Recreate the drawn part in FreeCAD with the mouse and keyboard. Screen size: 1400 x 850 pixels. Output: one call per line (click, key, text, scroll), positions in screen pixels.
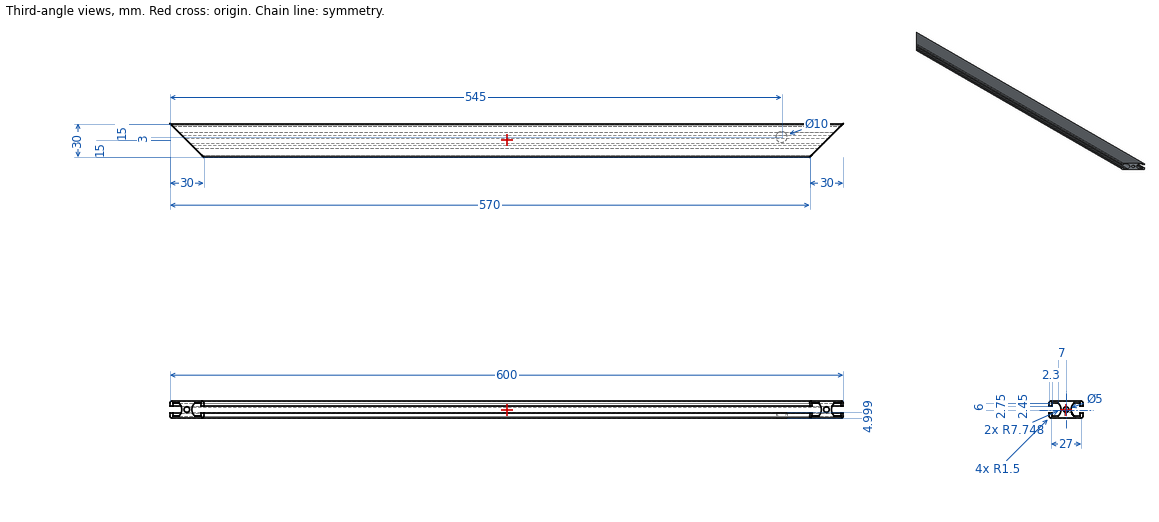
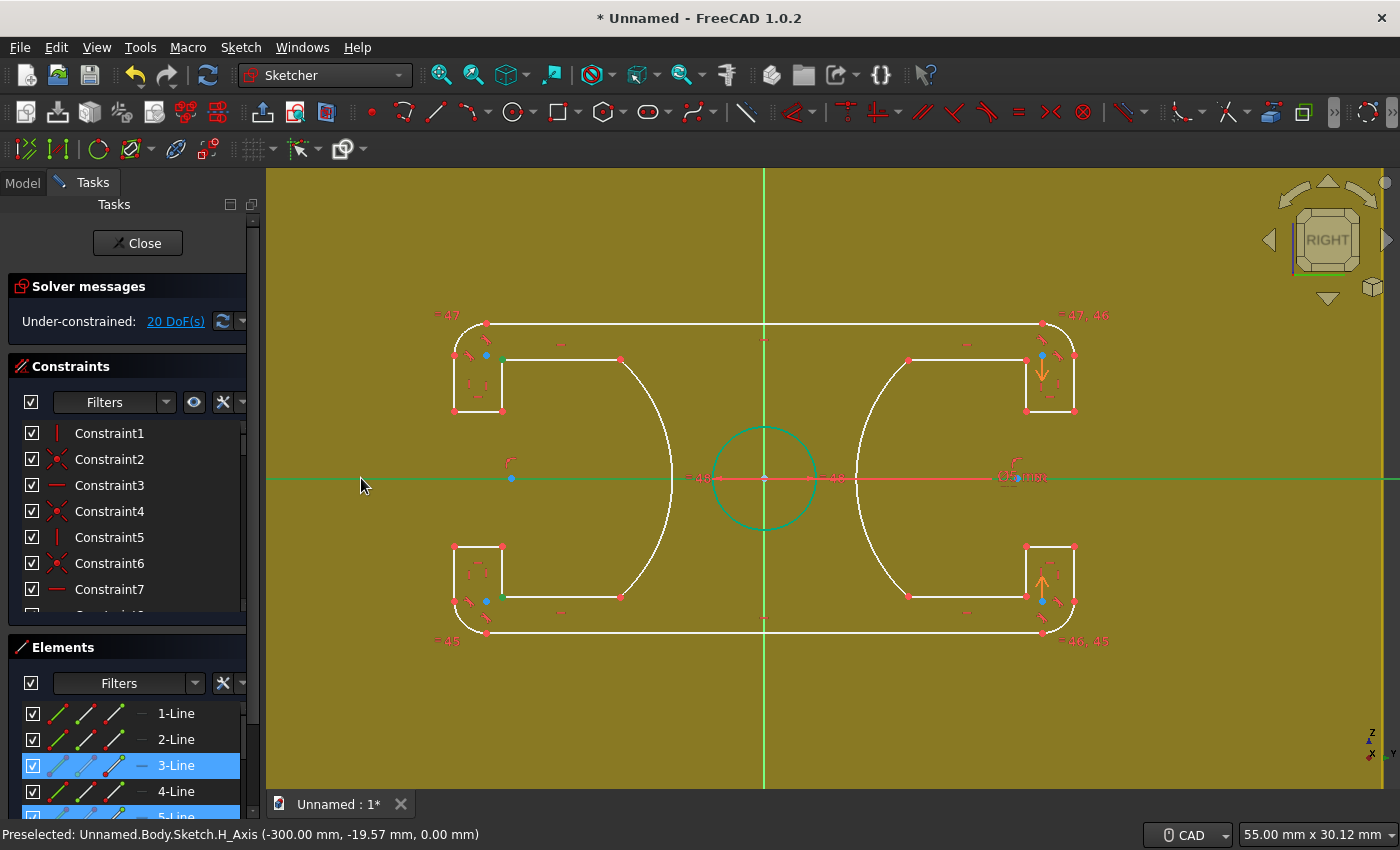
key(s)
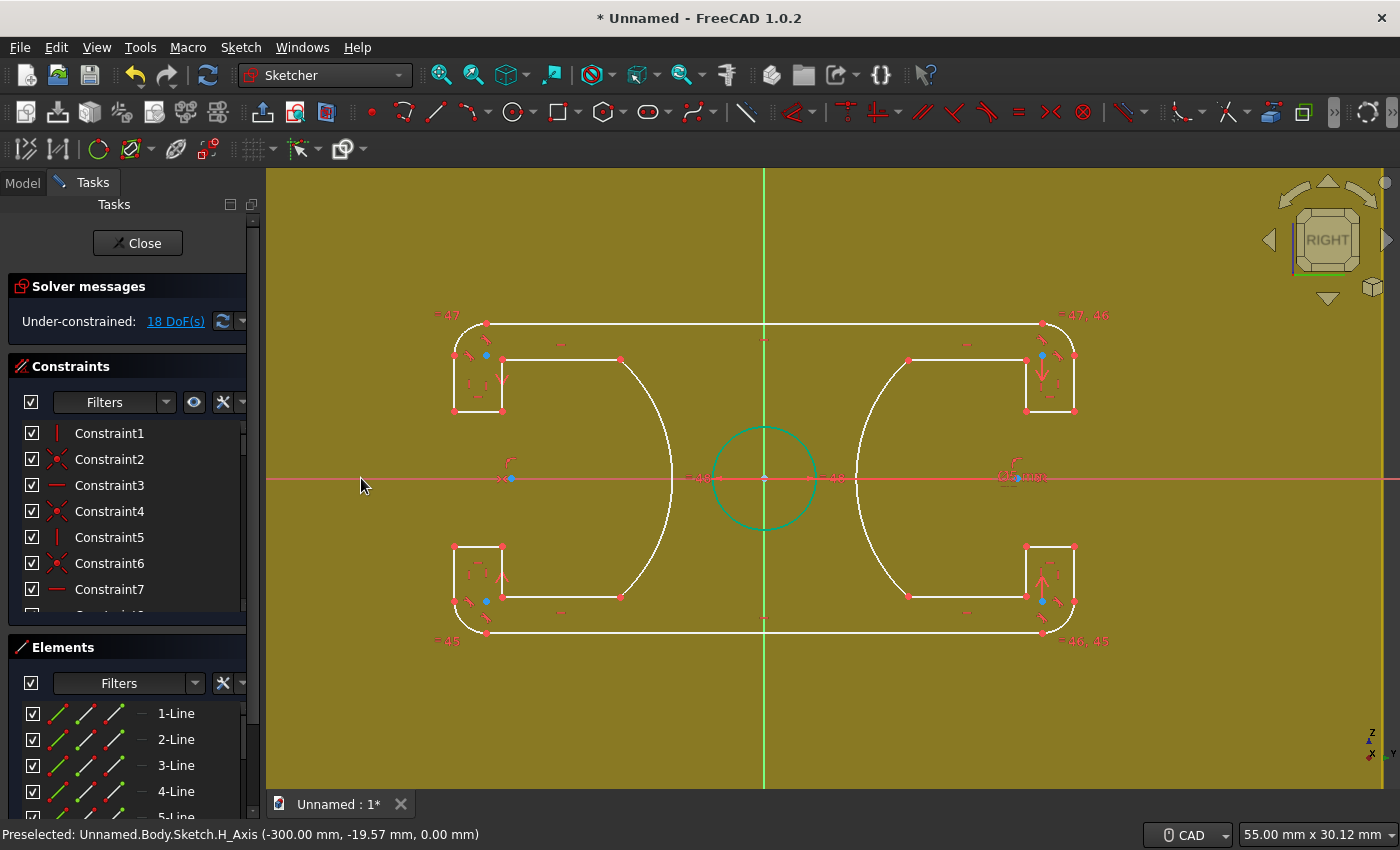
click(454, 412)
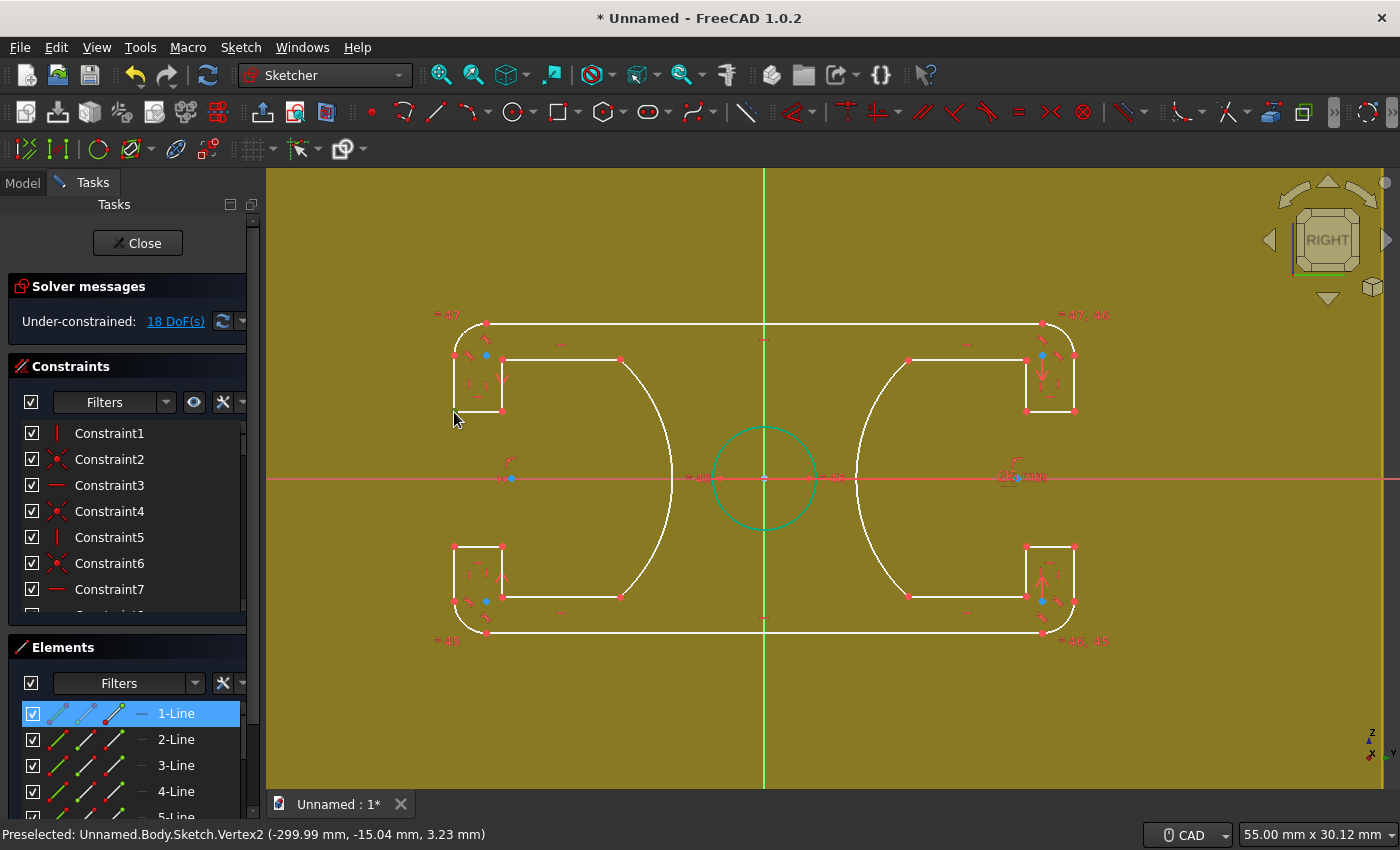
click(454, 547)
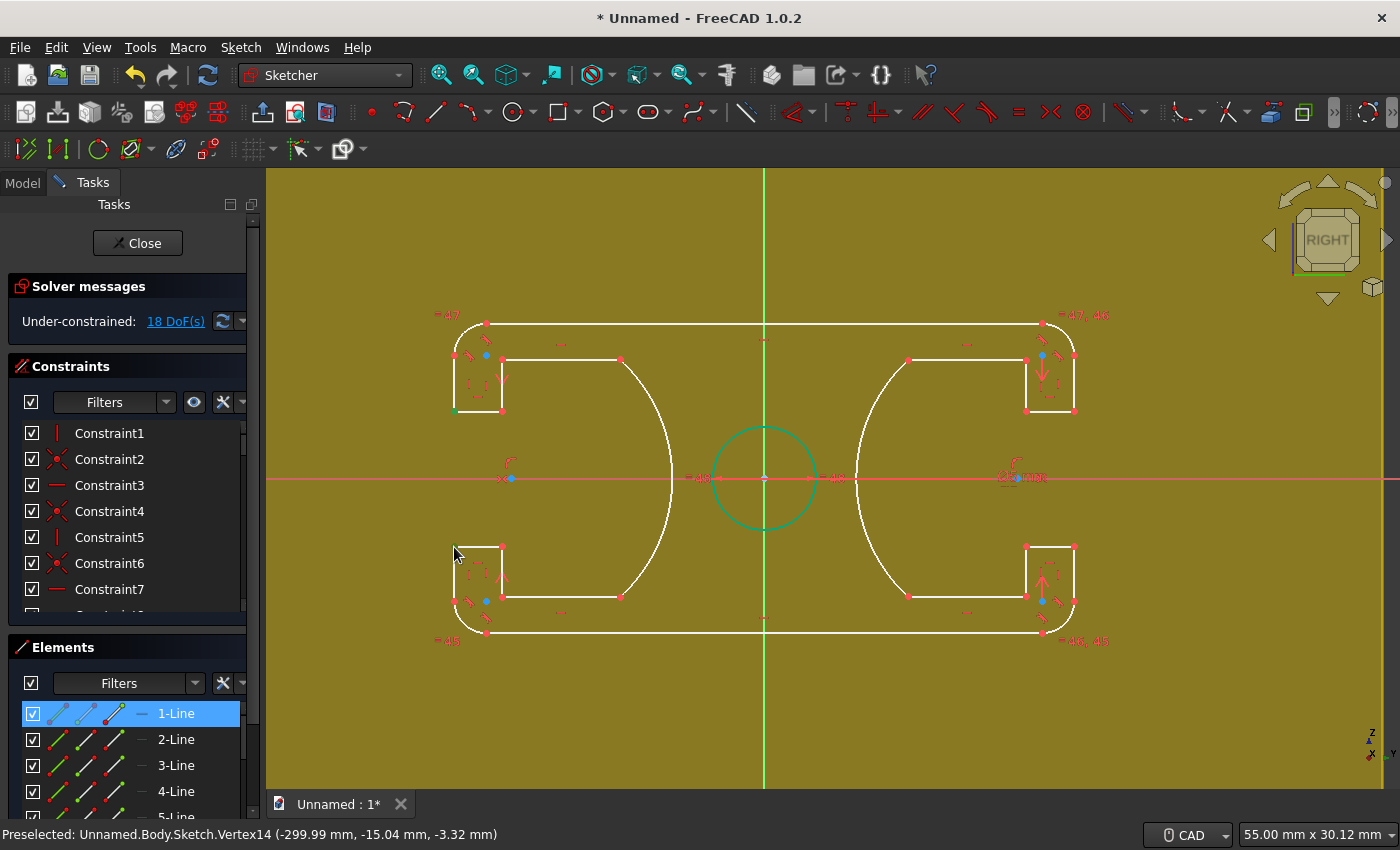
click(361, 478)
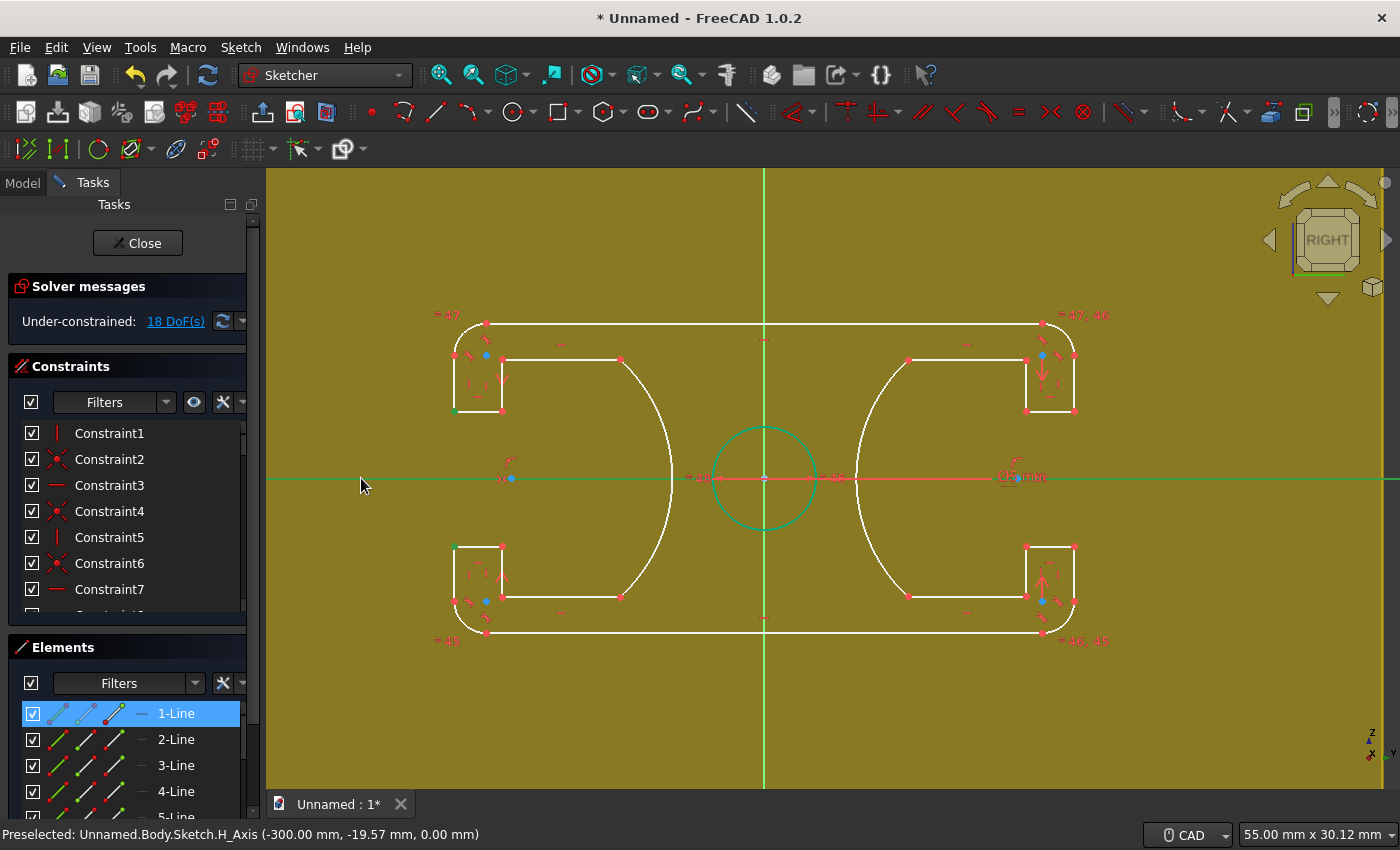
click(1052, 112)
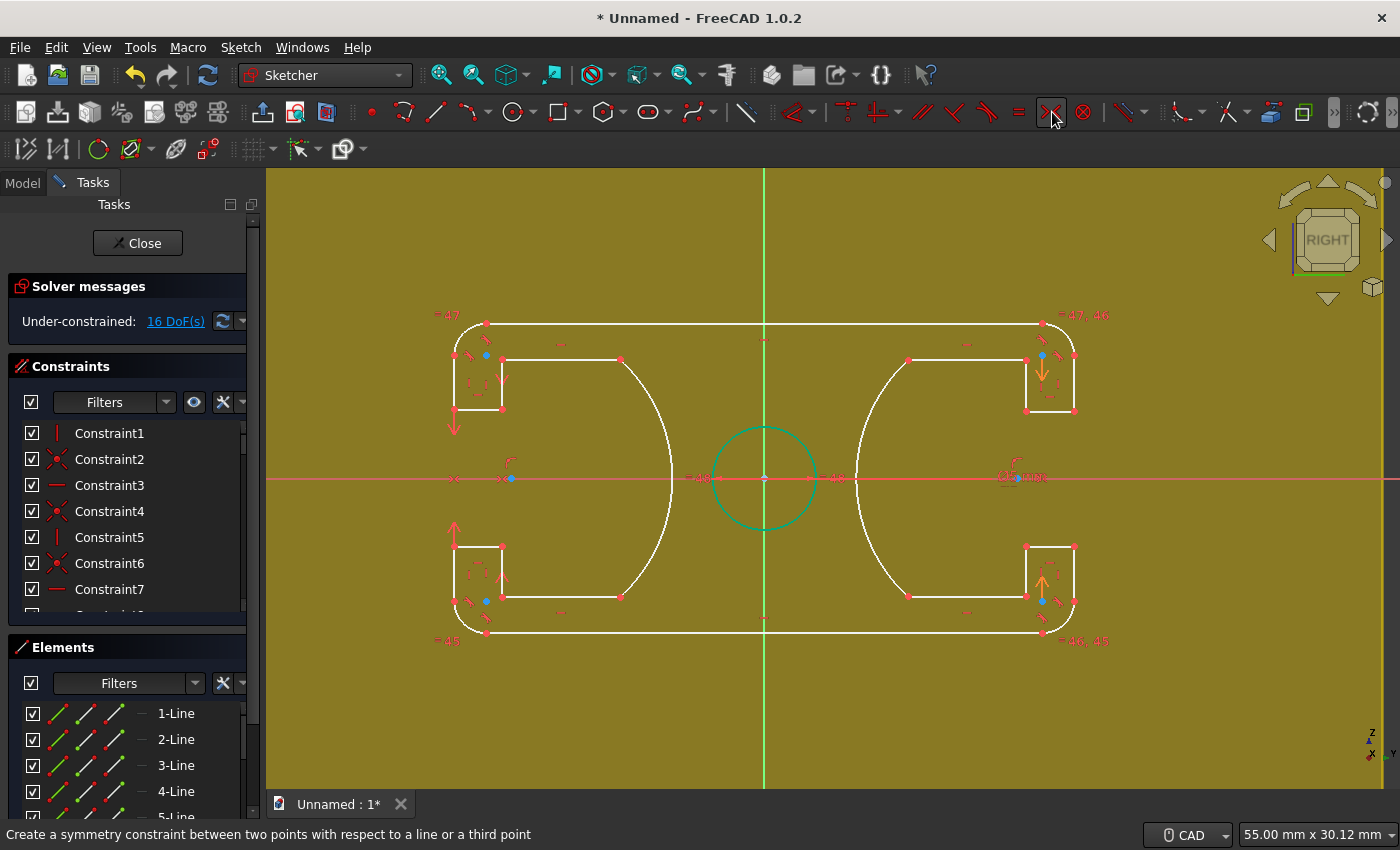
click(454, 547)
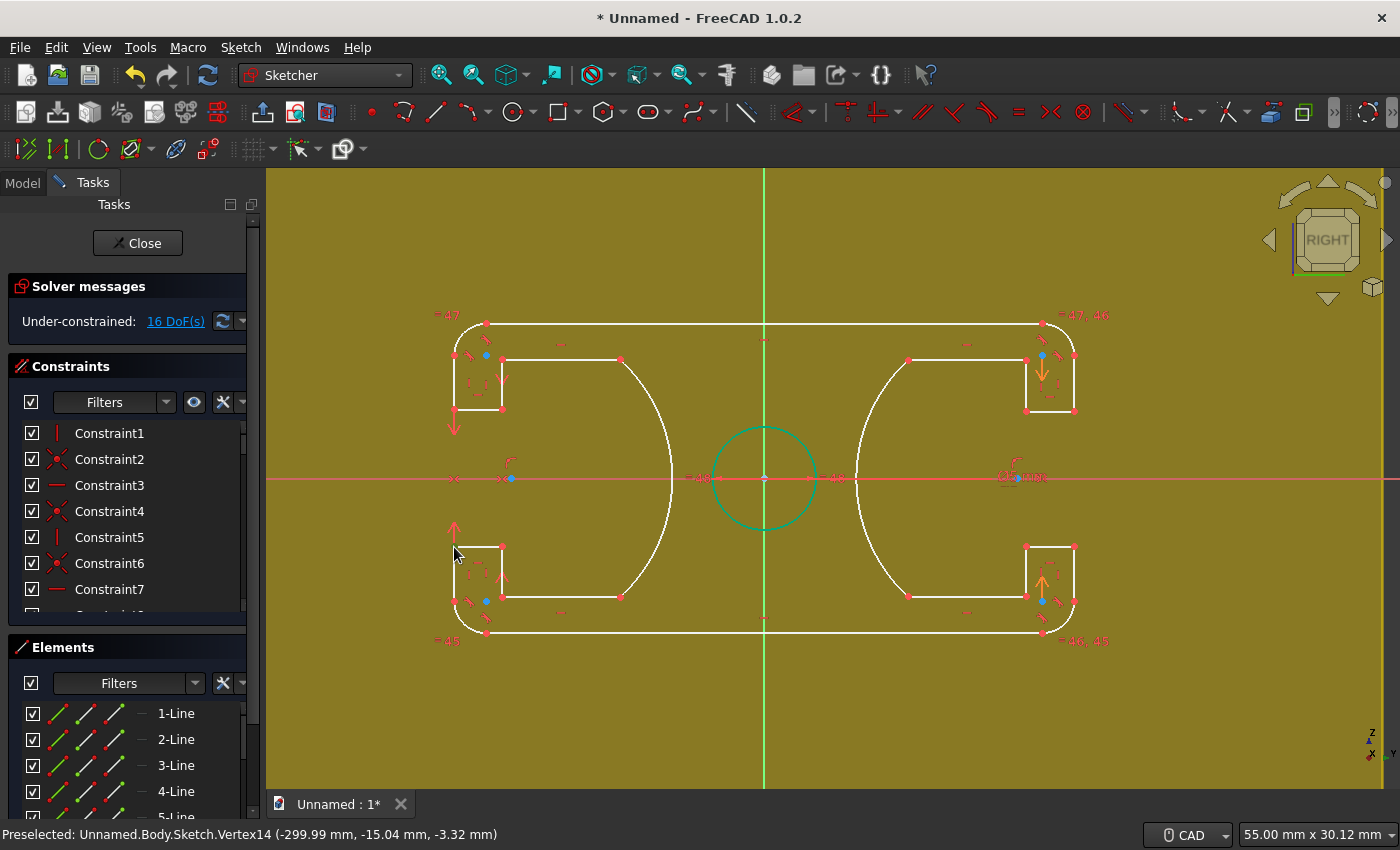
click(1074, 547)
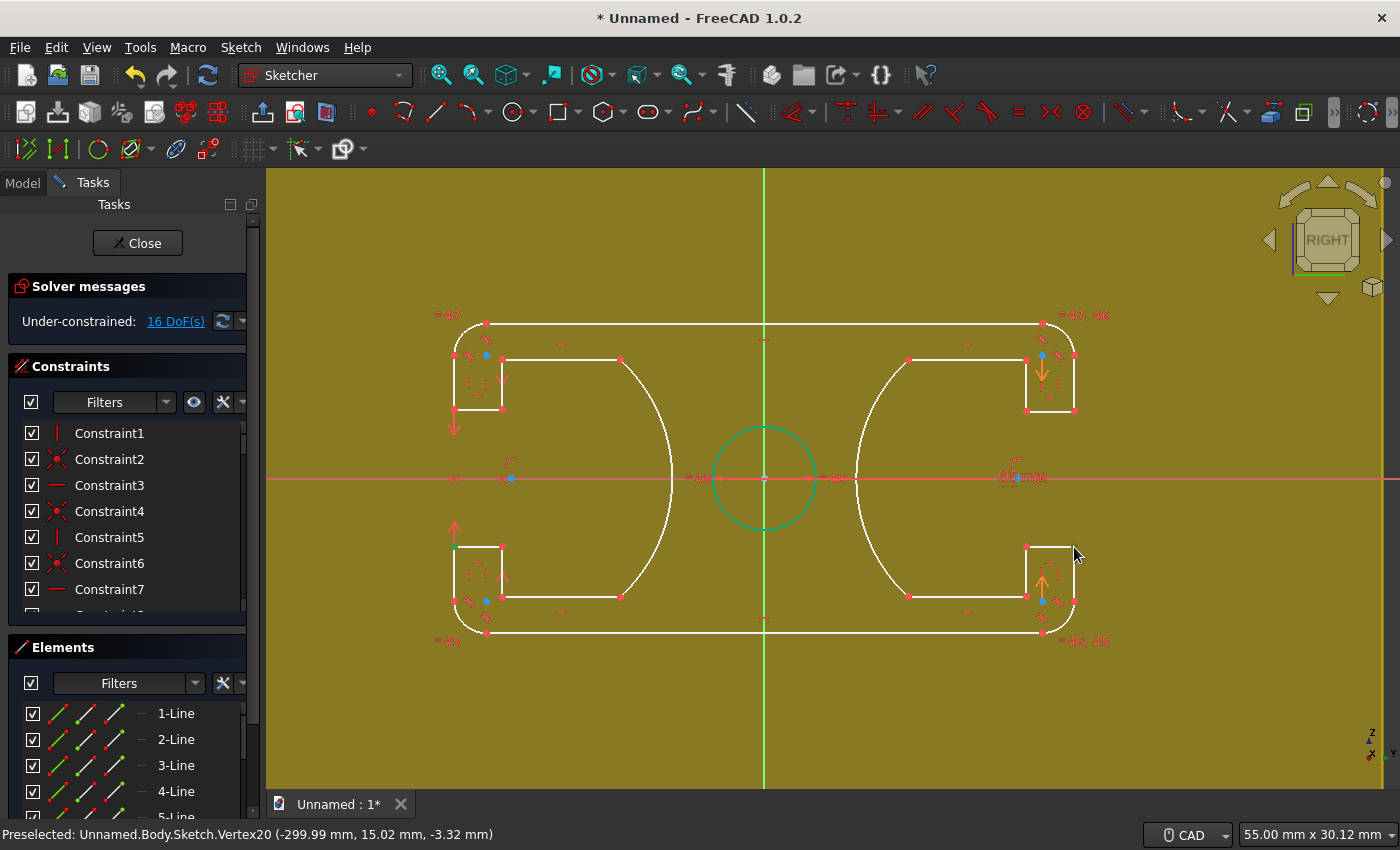
click(764, 721)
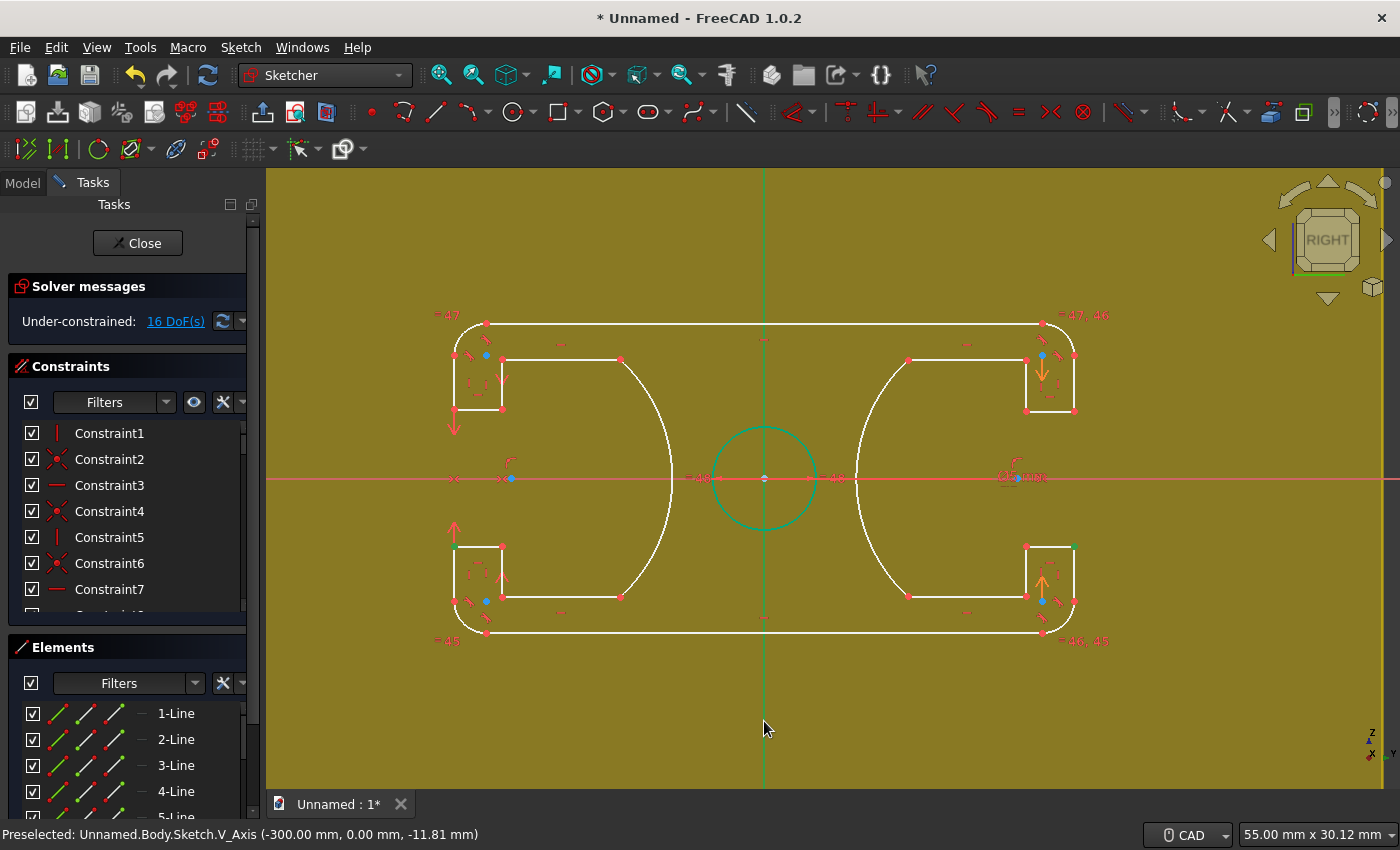
key(s)